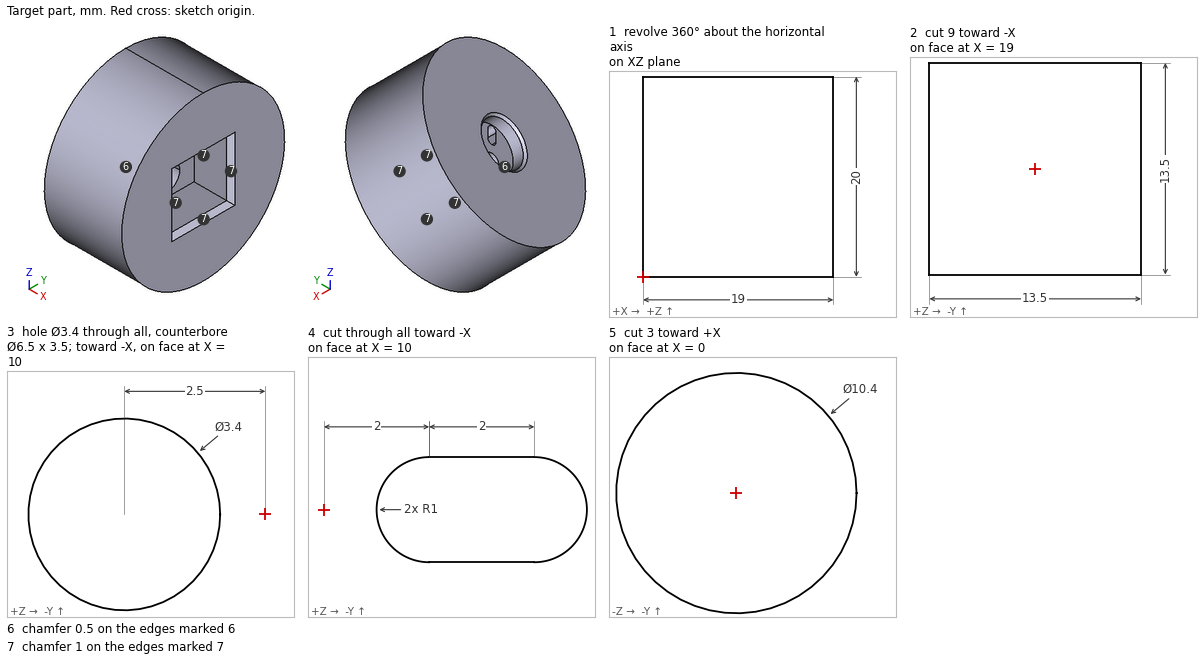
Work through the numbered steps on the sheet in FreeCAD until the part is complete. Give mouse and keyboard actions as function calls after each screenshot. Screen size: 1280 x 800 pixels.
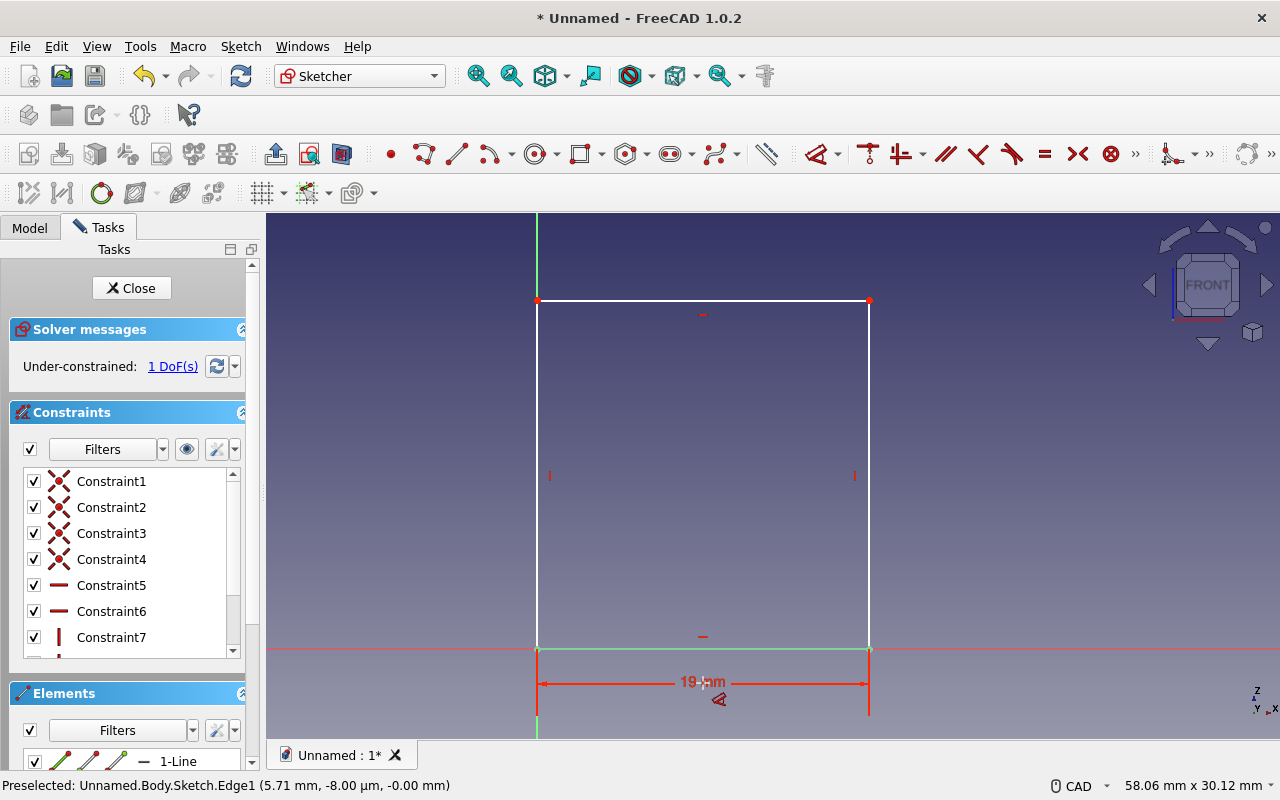
click(869, 545)
click(903, 475)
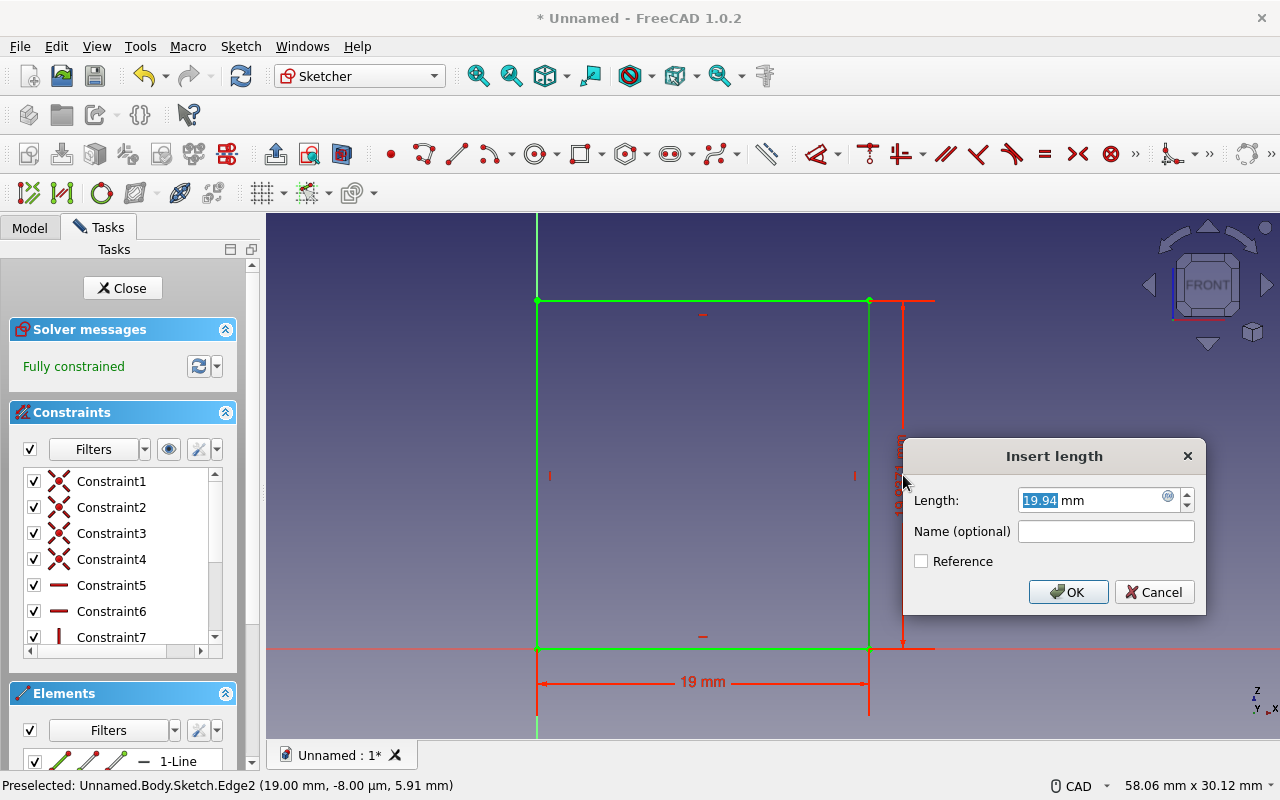
text(20)
key(Return)
key(Escape)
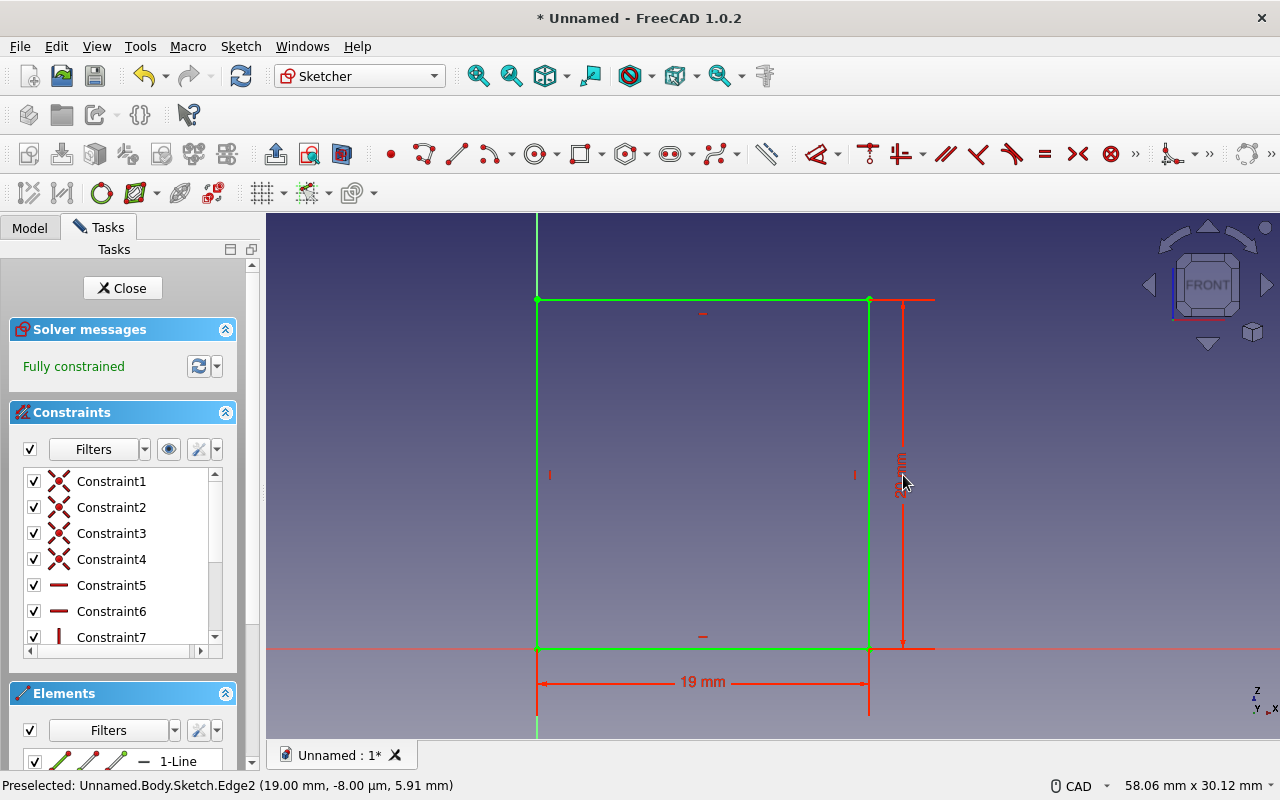
click(123, 288)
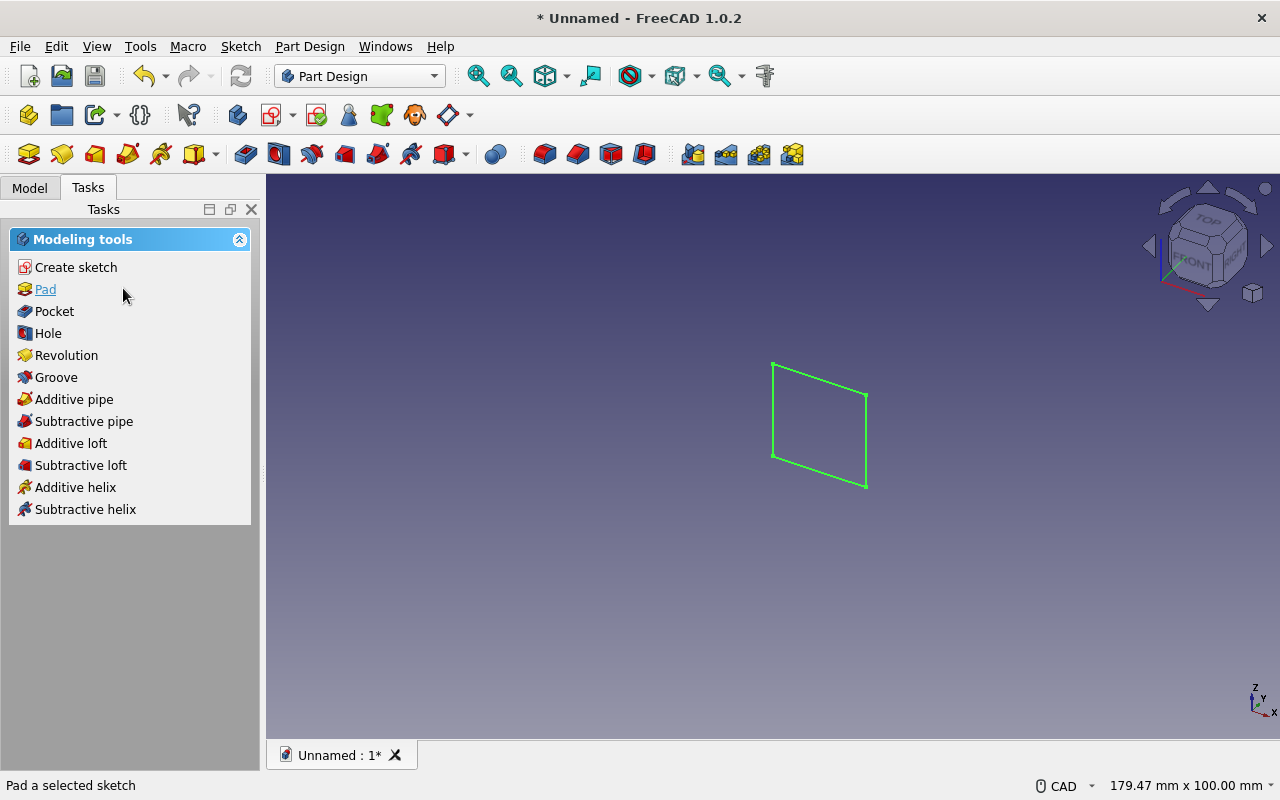
click(62, 154)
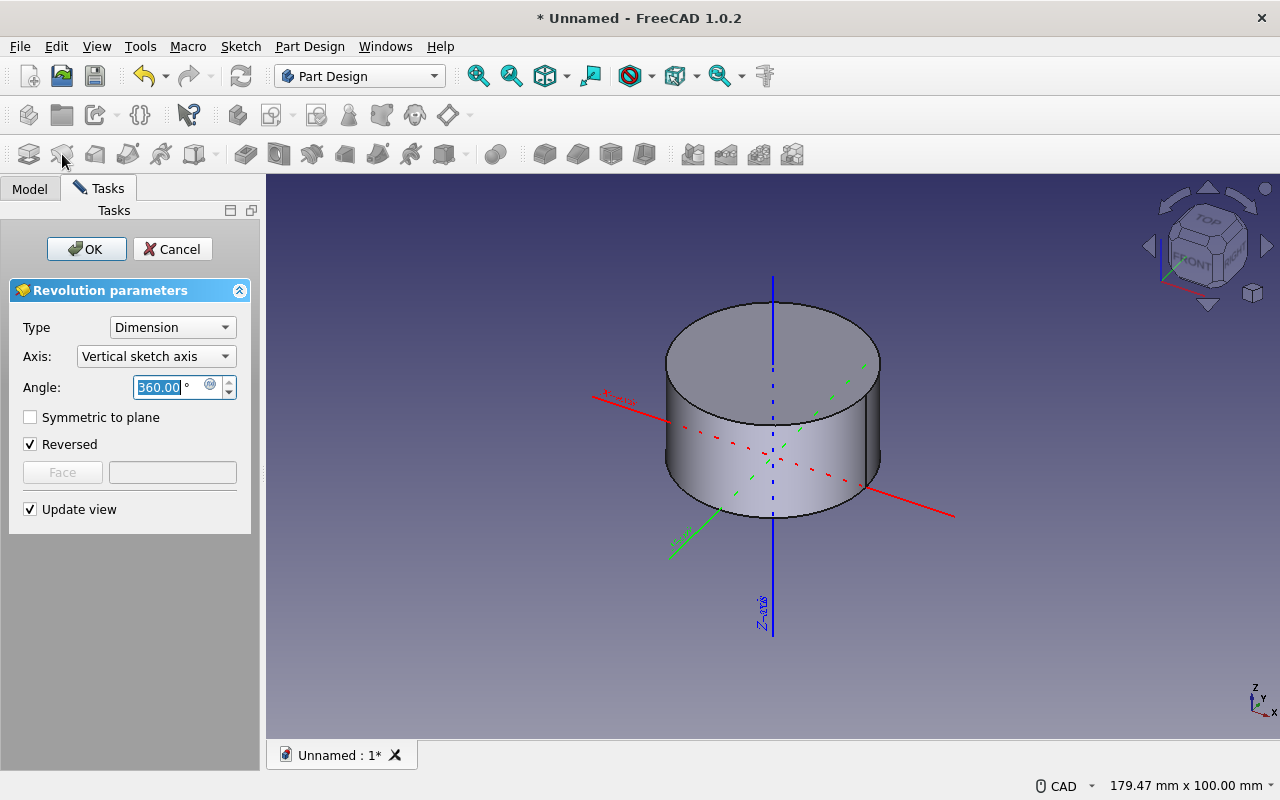
click(157, 356)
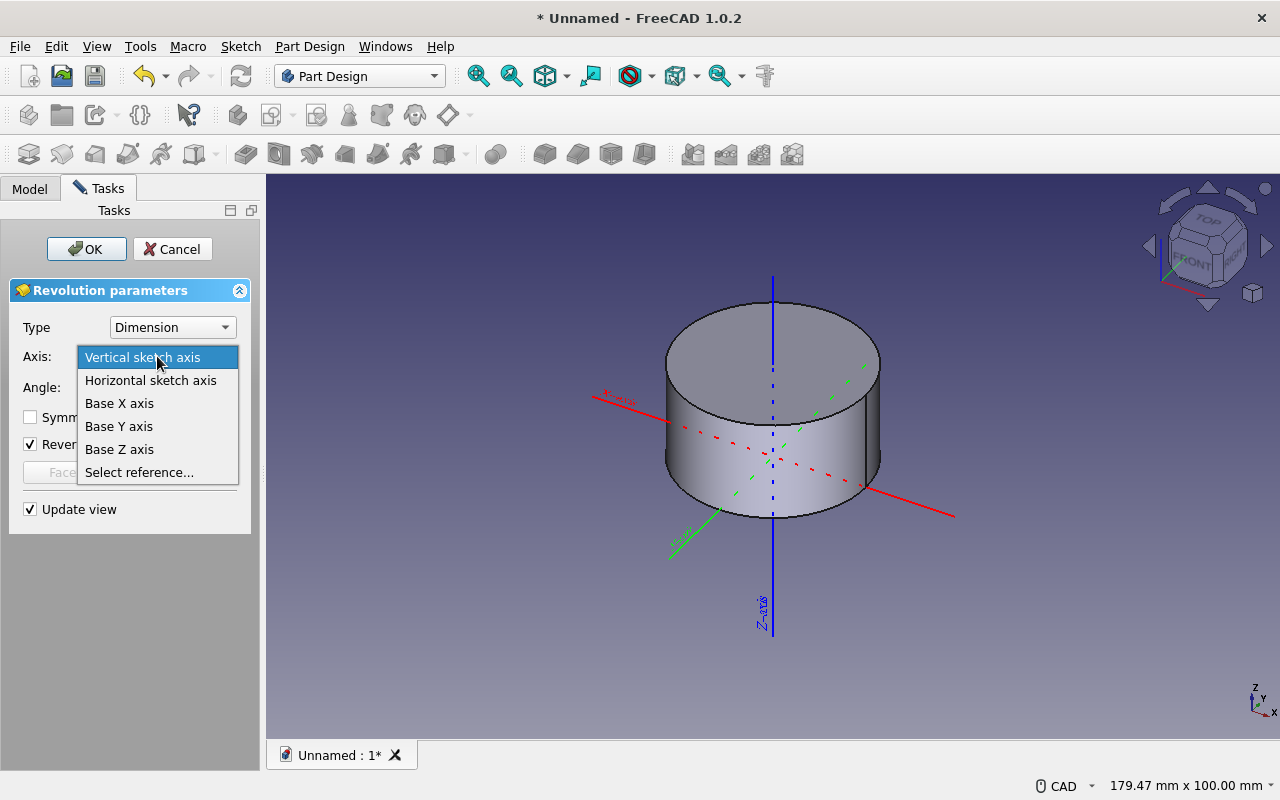
click(156, 380)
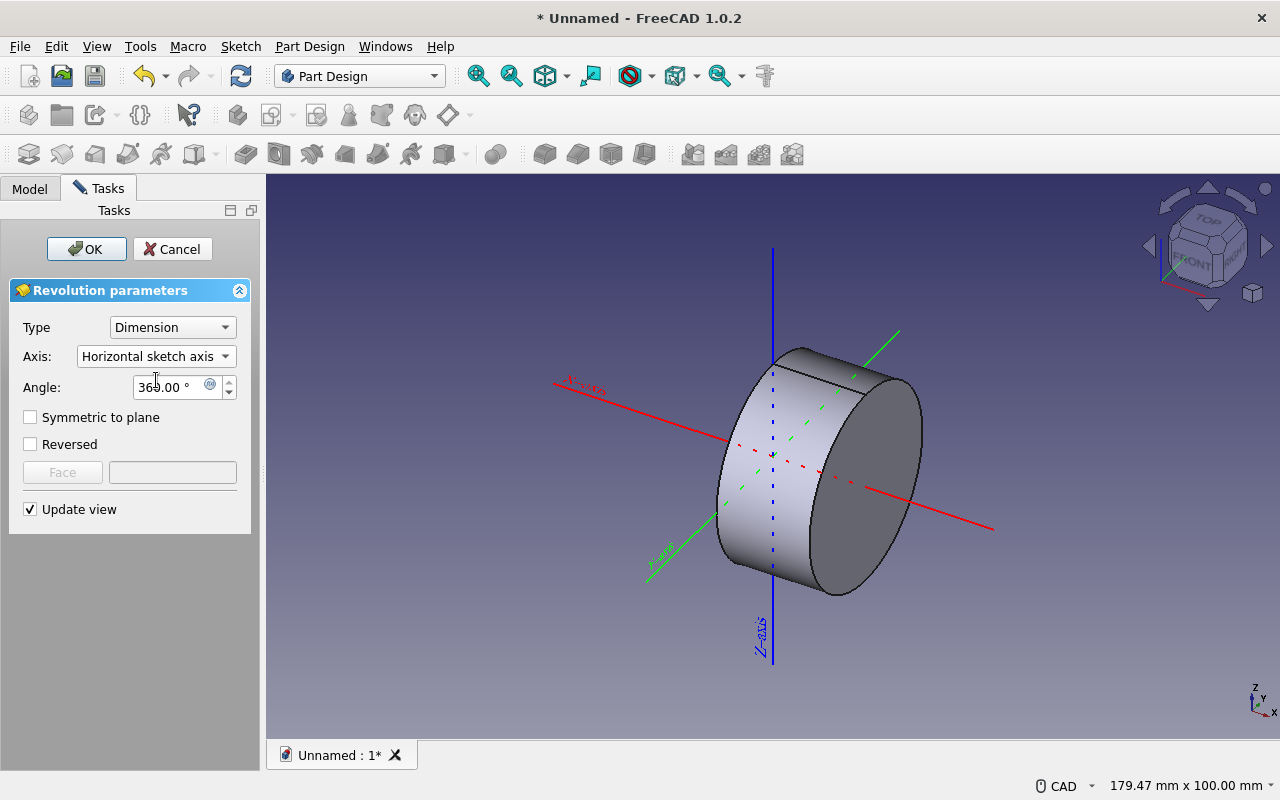
click(87, 249)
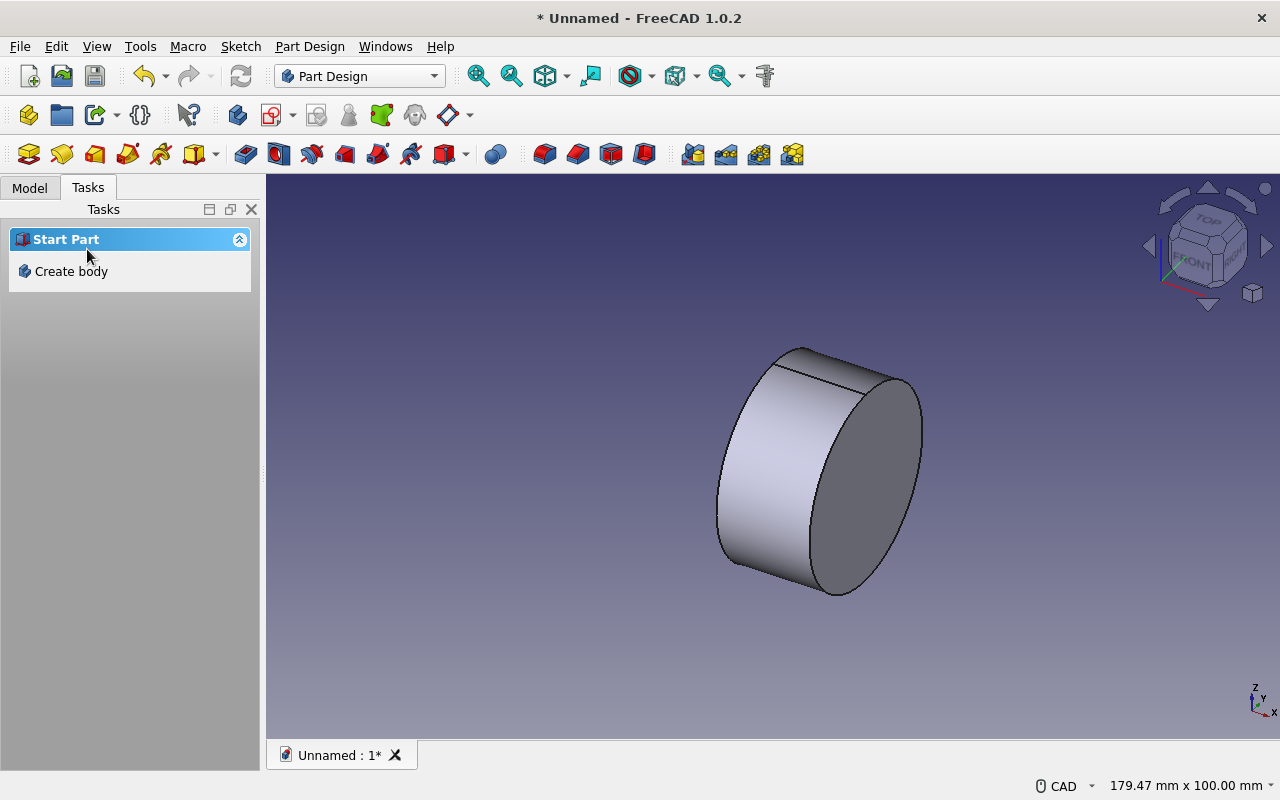
click(866, 486)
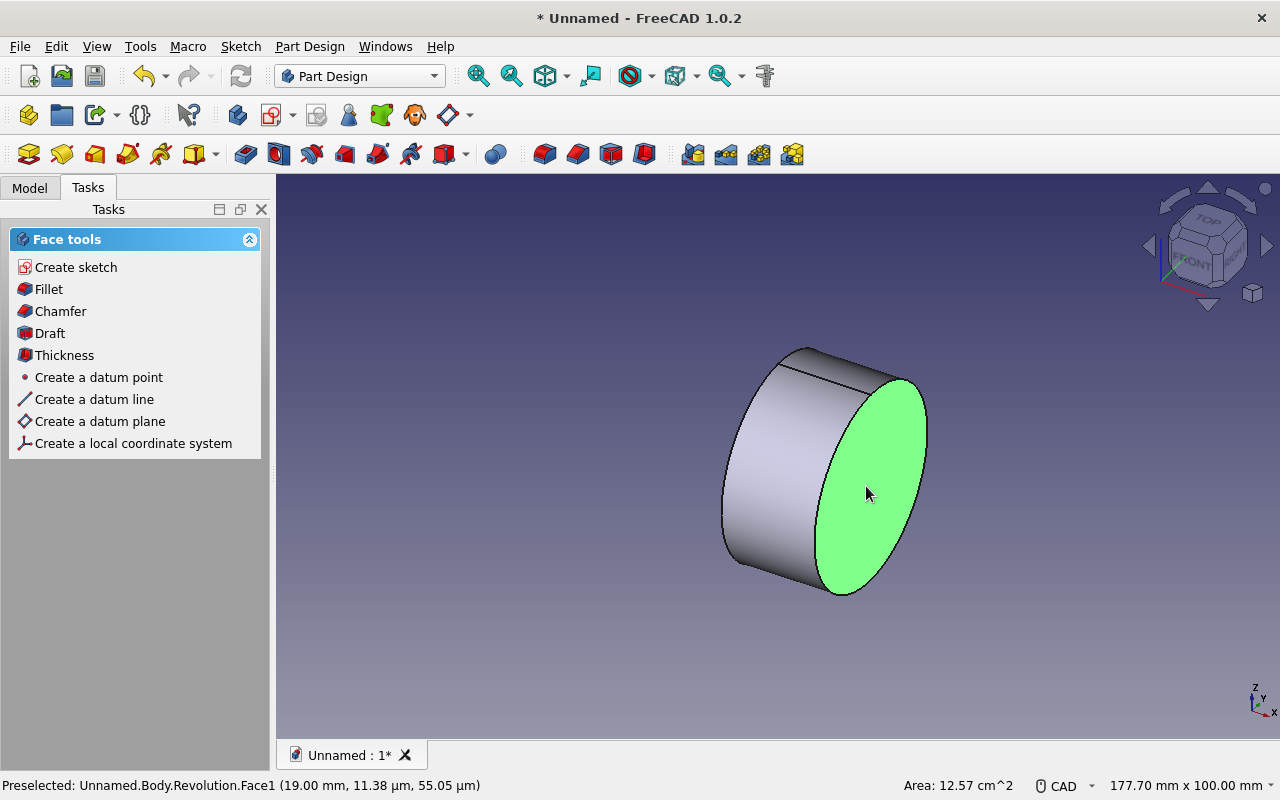
click(270, 116)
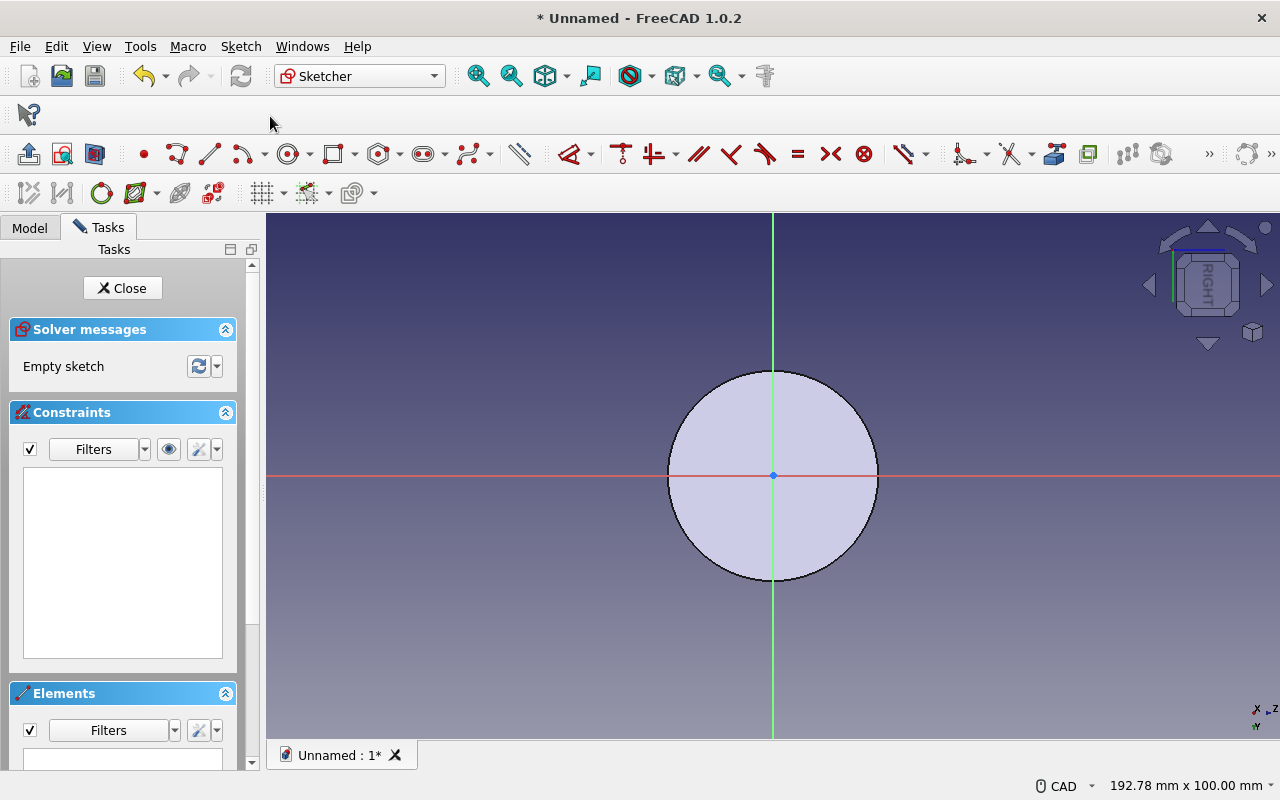
scroll(790, 476, up, 8)